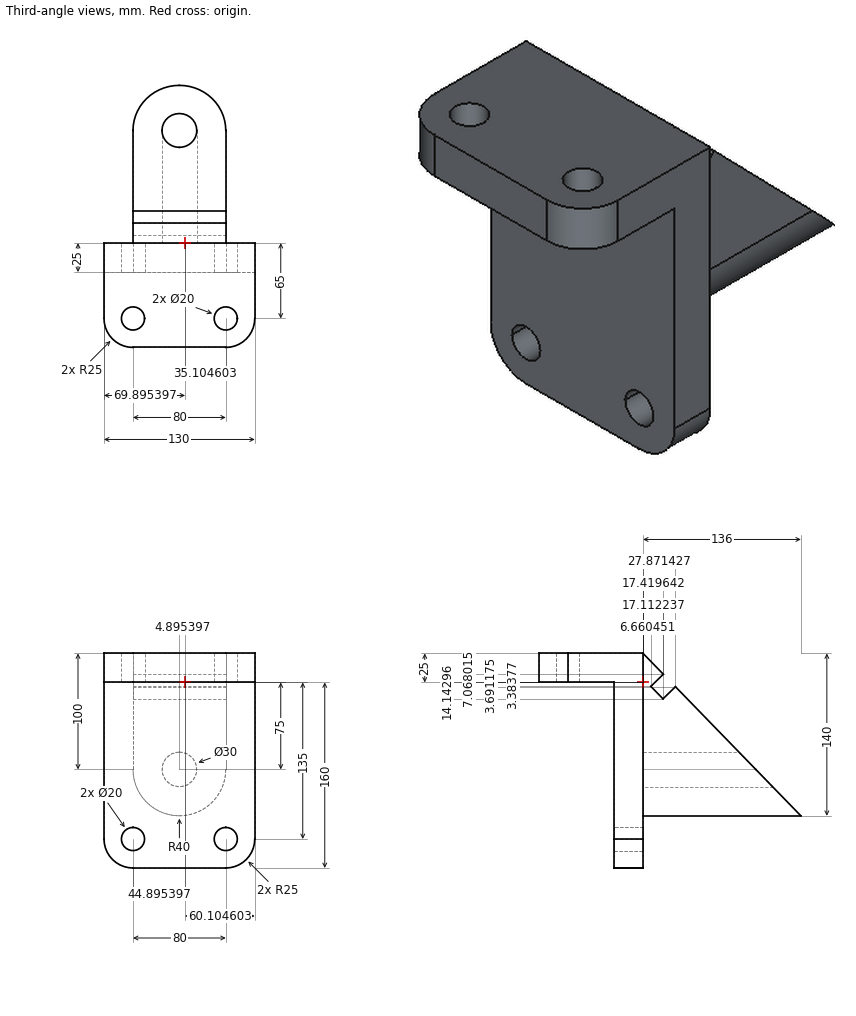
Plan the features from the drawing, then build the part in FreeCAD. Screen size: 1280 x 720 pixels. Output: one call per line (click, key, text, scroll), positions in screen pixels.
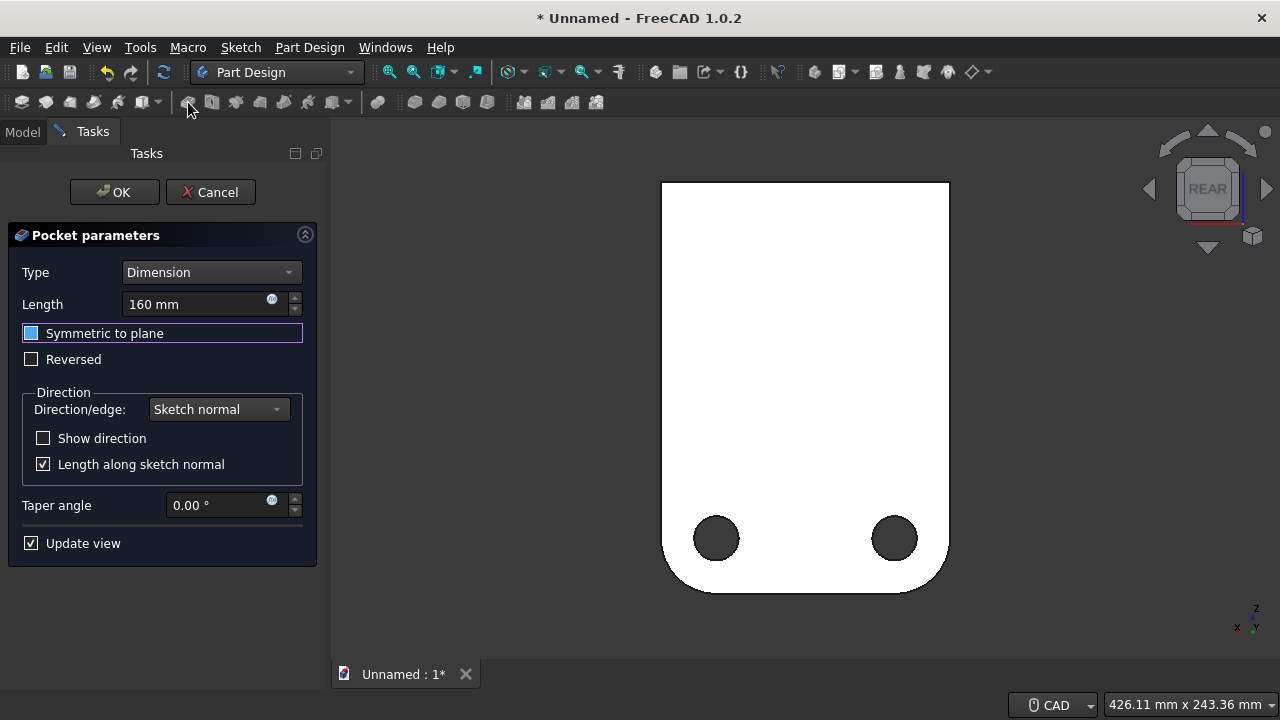
click(115, 192)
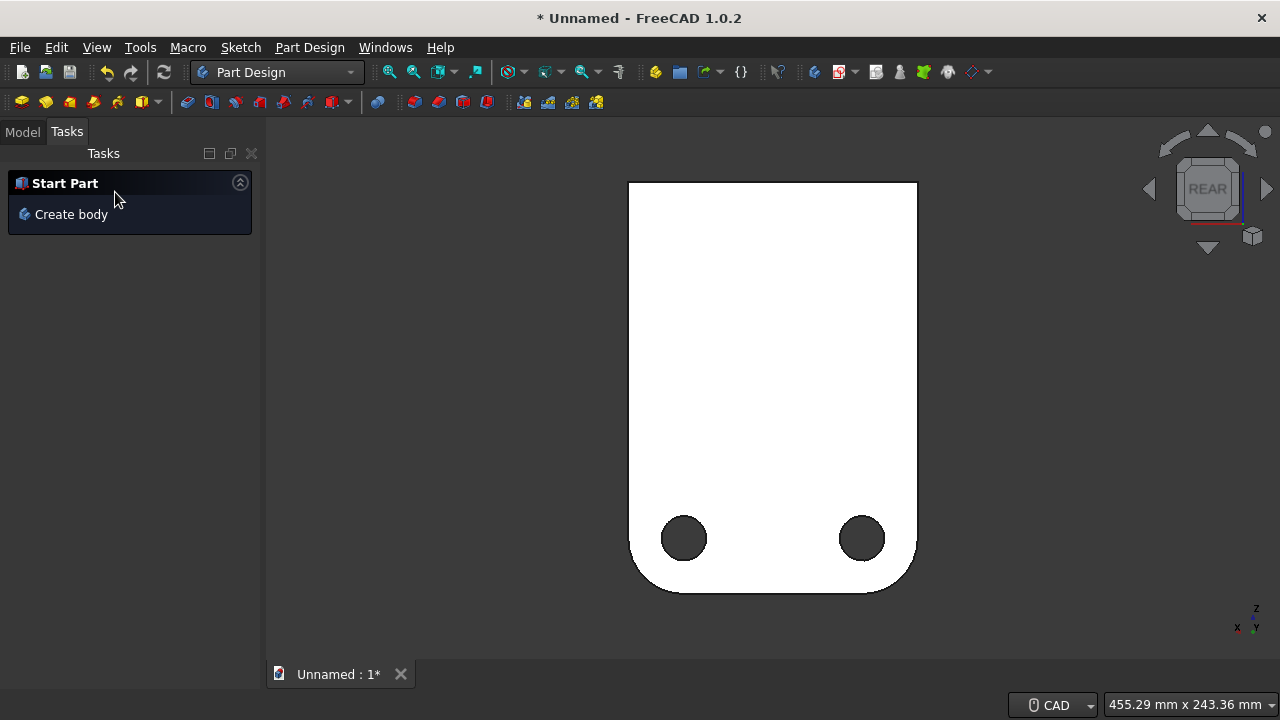
click(773, 328)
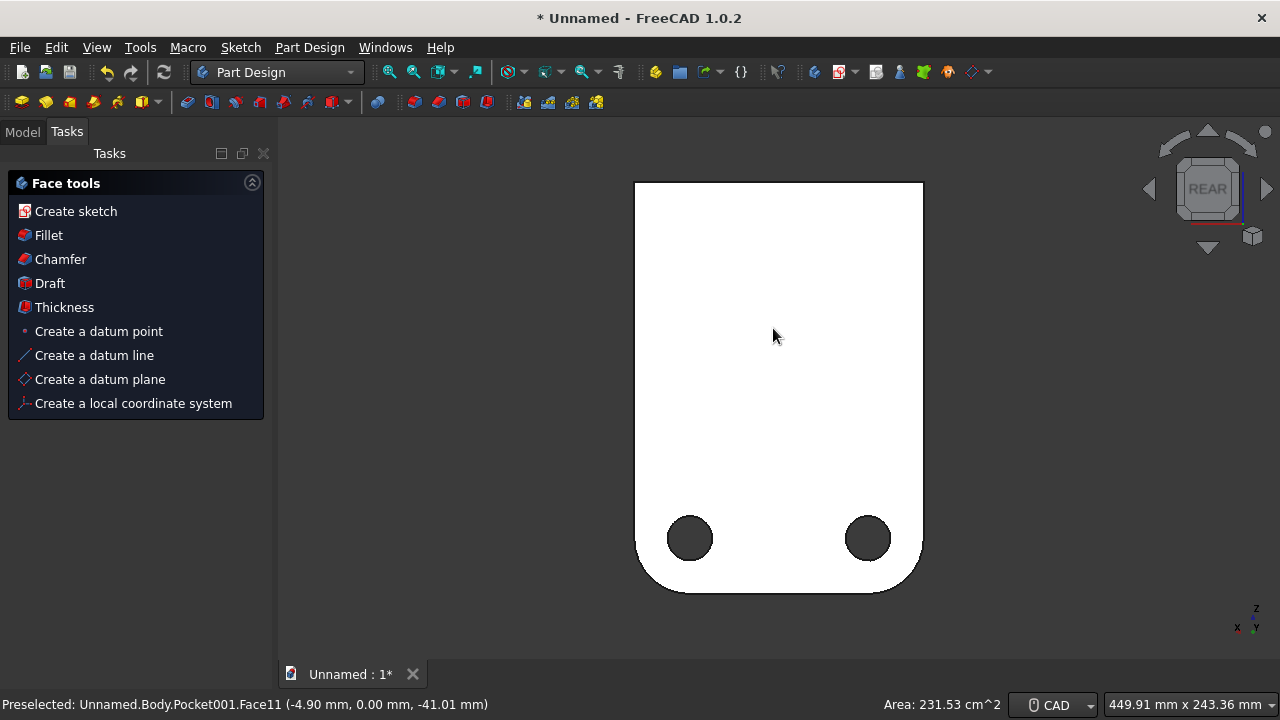
click(840, 72)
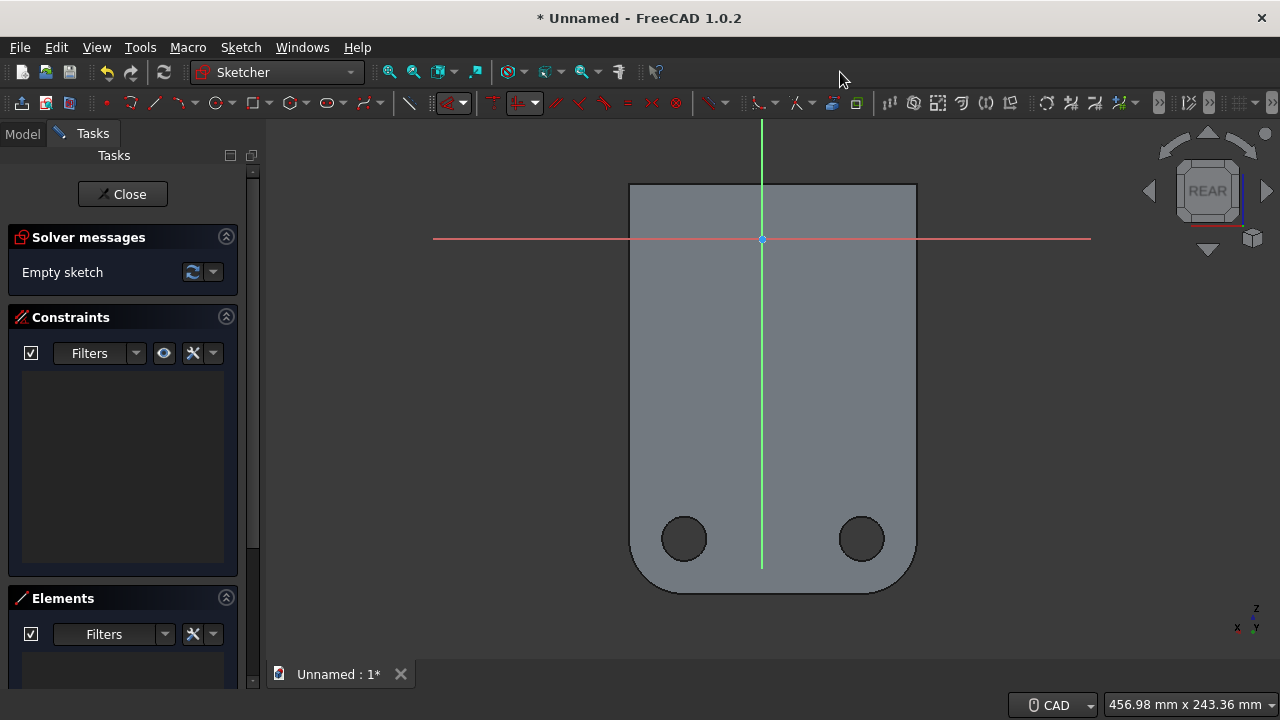
click(132, 104)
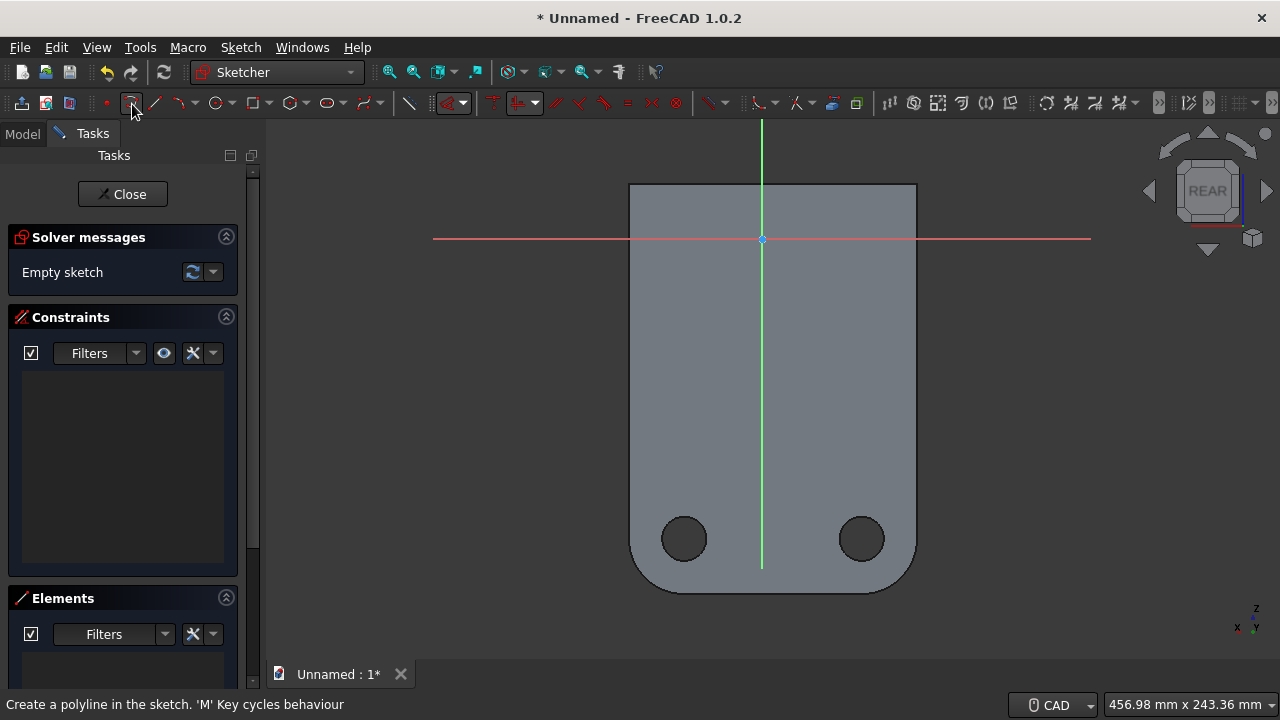
click(862, 406)
click(862, 184)
click(684, 184)
click(684, 406)
right_click(684, 406)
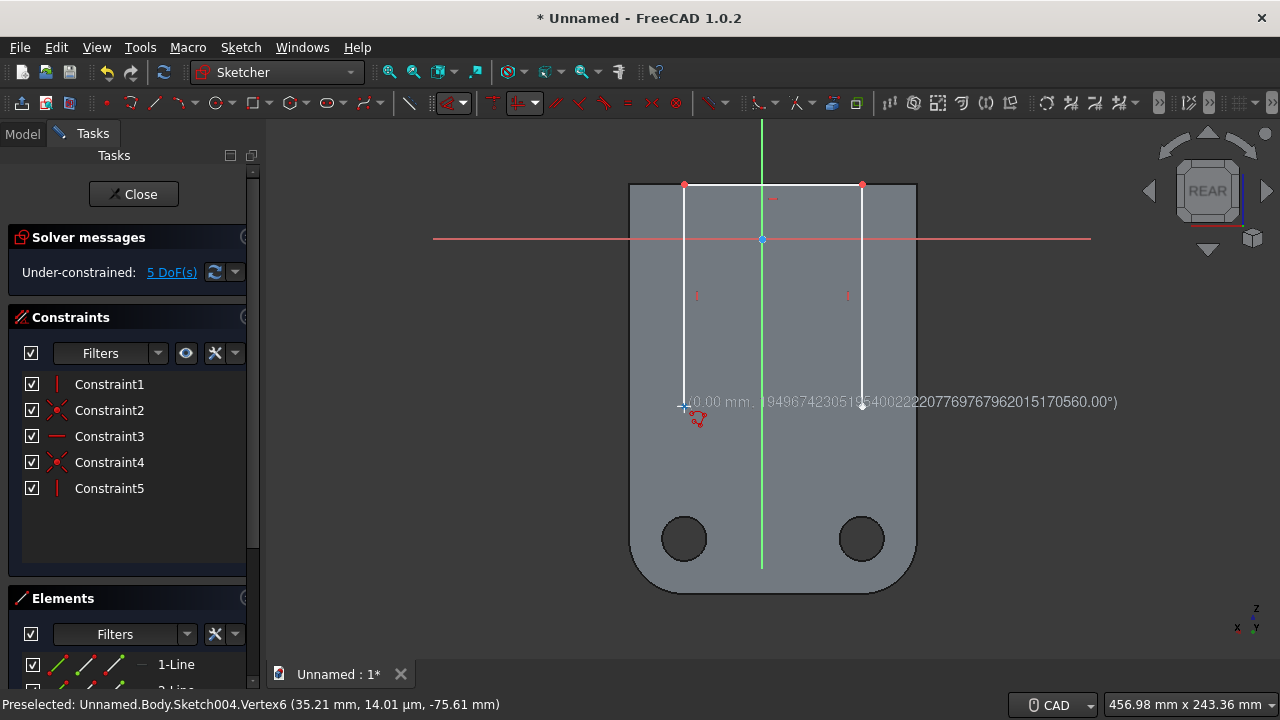
click(180, 104)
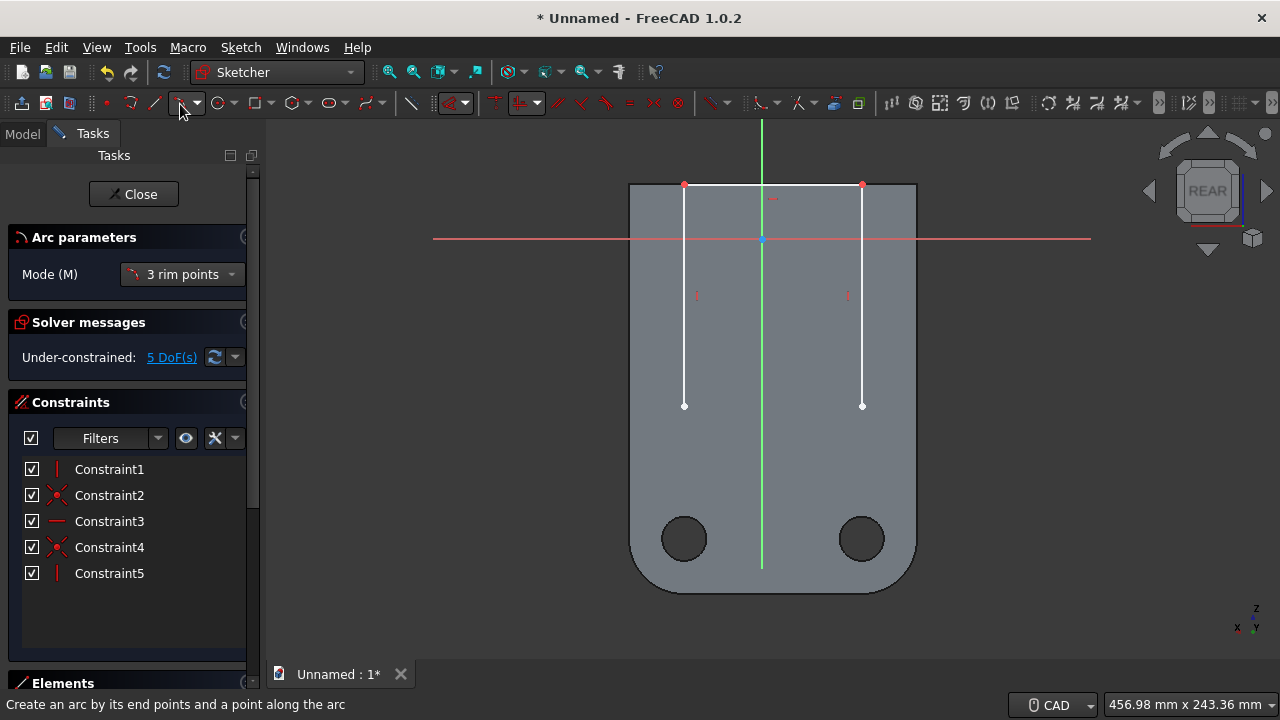
click(684, 407)
click(862, 407)
click(746, 490)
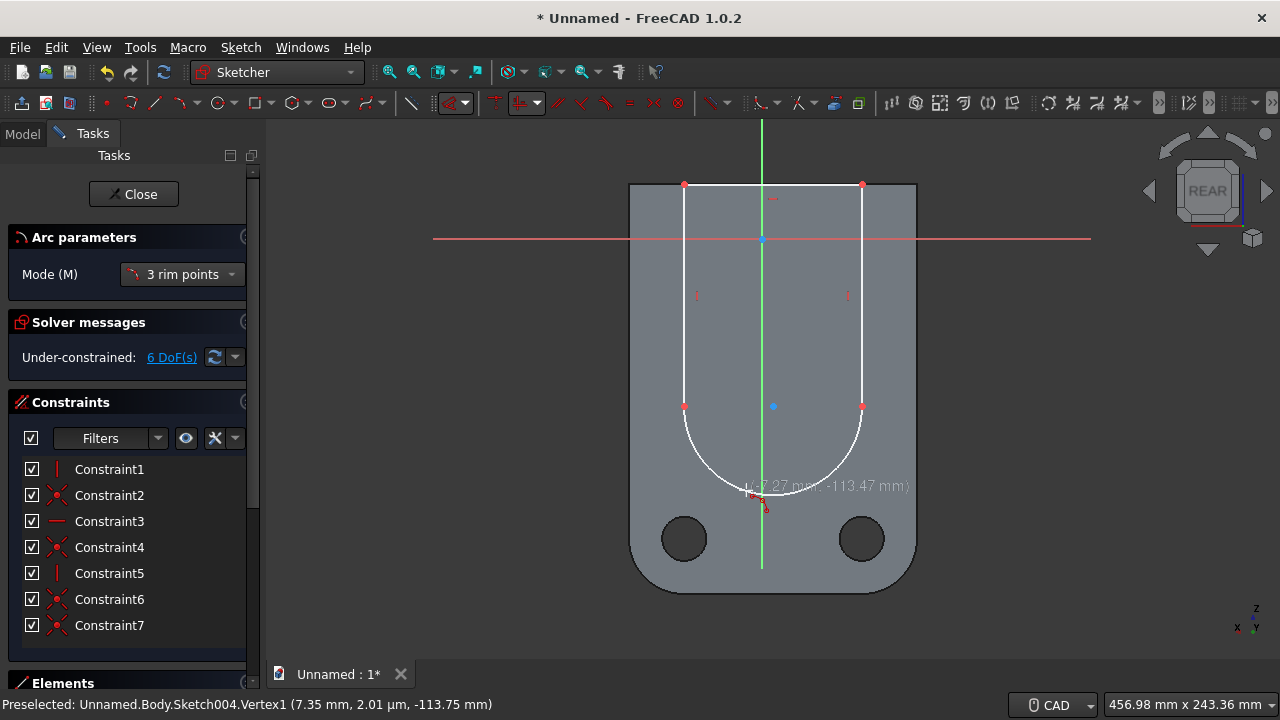
click(218, 104)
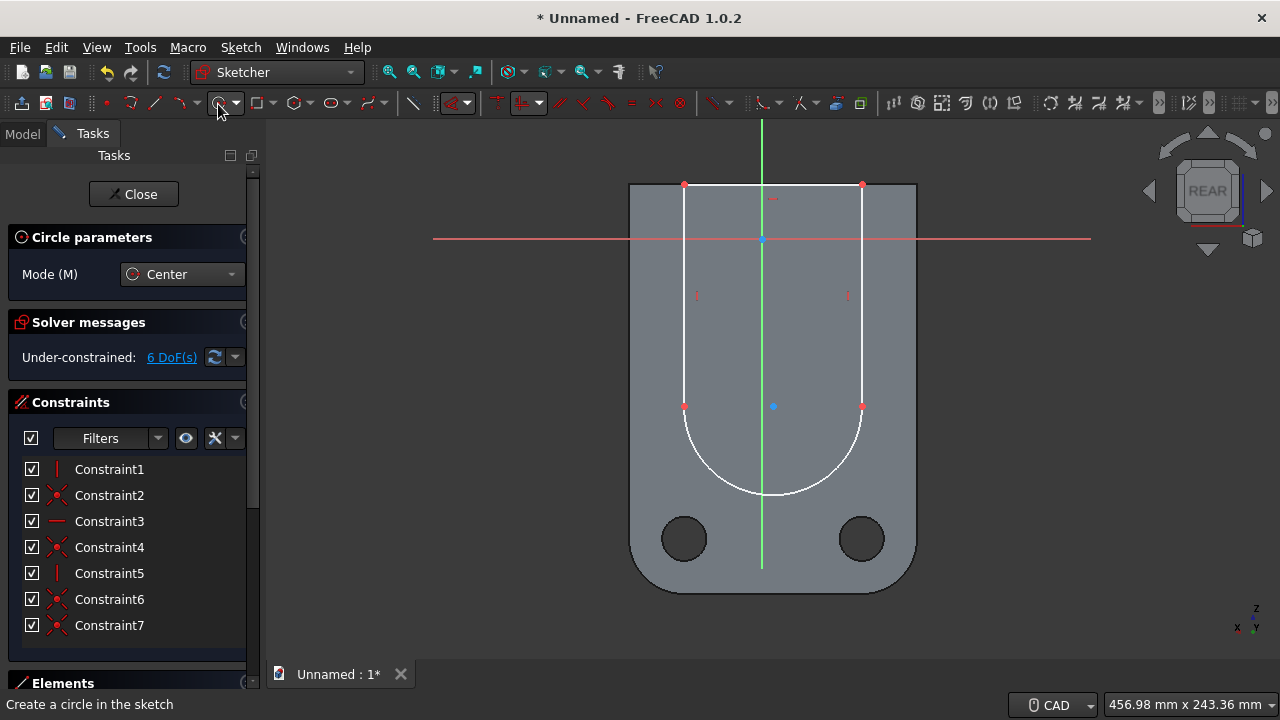
scroll(773, 406, up, 2)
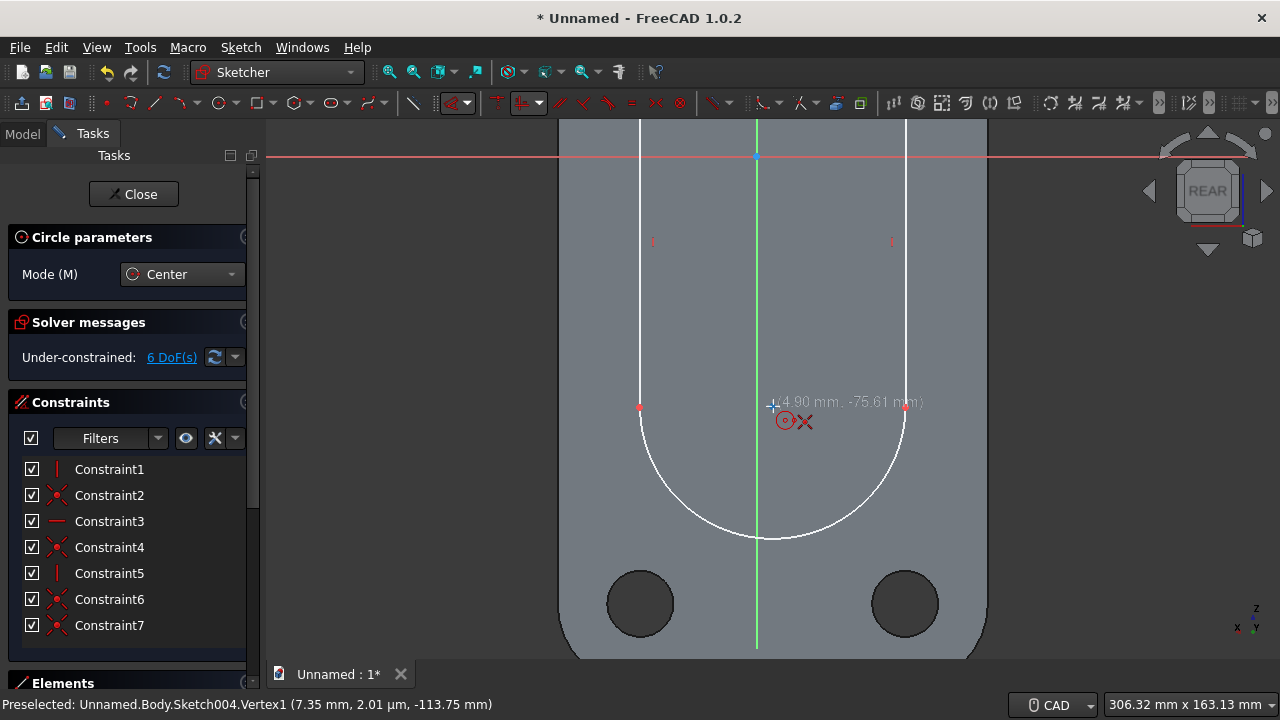
click(773, 405)
click(808, 370)
key(Escape)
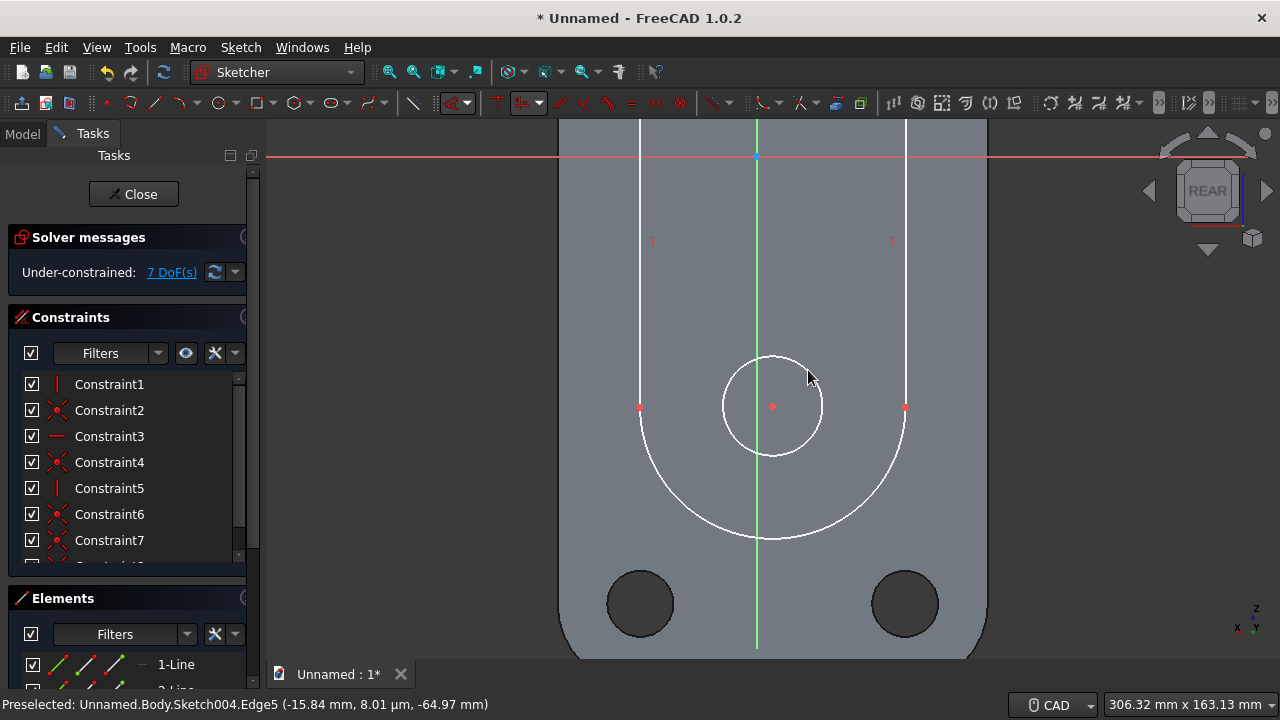
click(695, 514)